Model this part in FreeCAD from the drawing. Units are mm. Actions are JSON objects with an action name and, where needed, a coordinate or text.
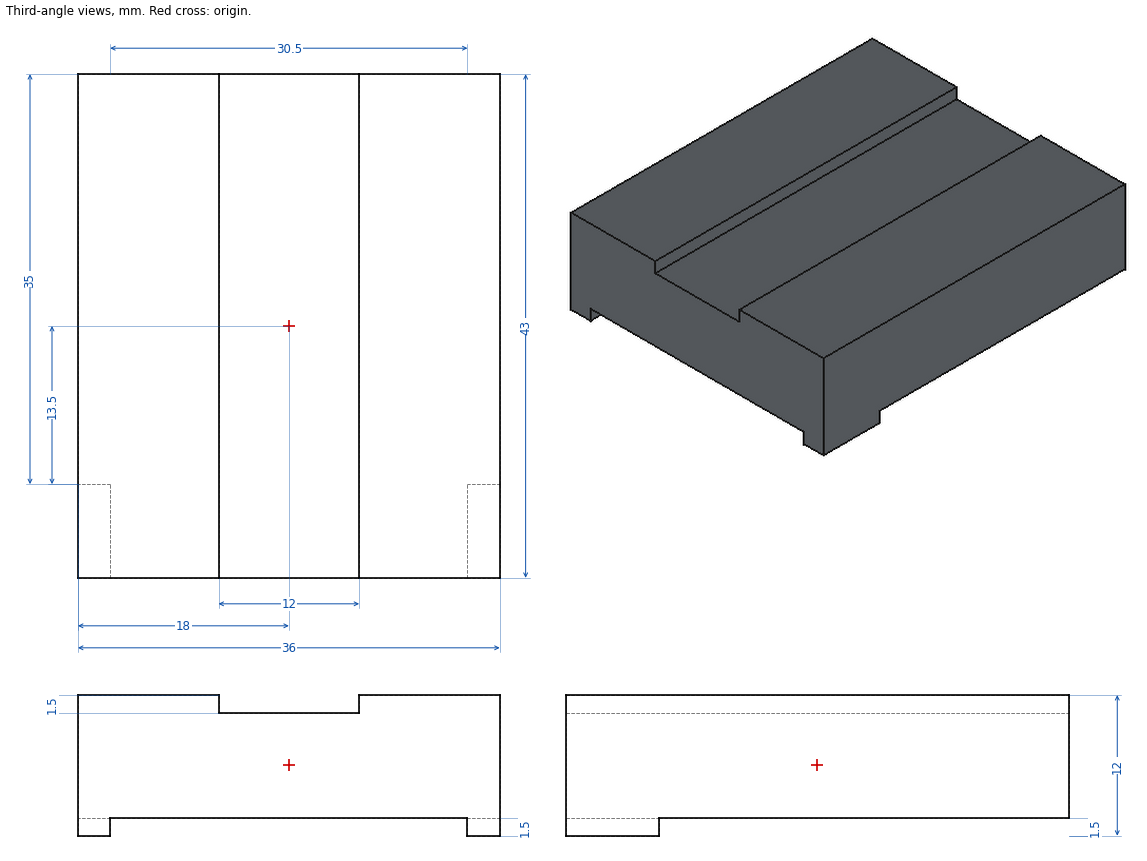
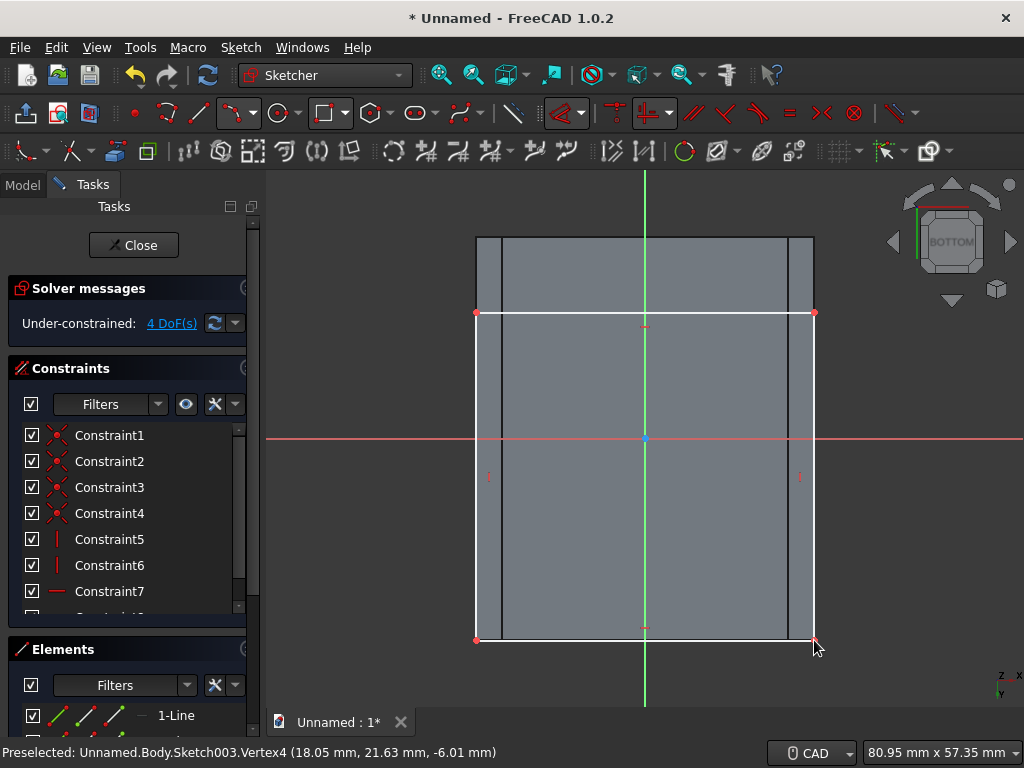
{"action": "key", "text": "d"}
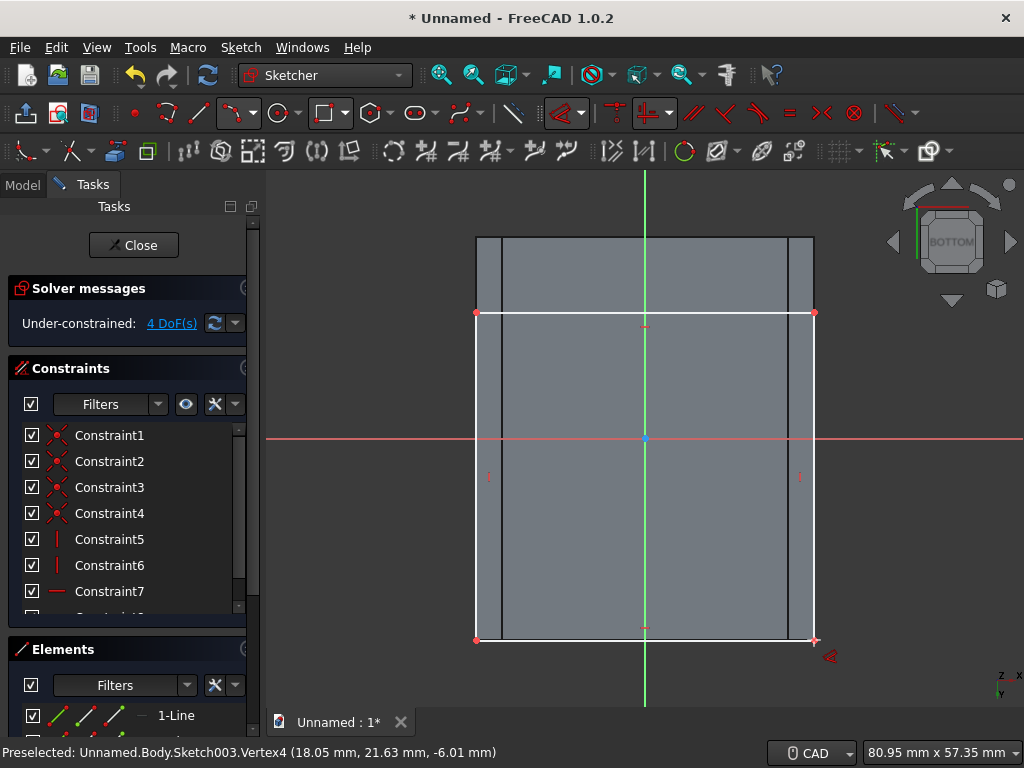
{"action": "left_click", "coordinate": [476, 411]}
{"action": "left_click", "coordinate": [442, 477]}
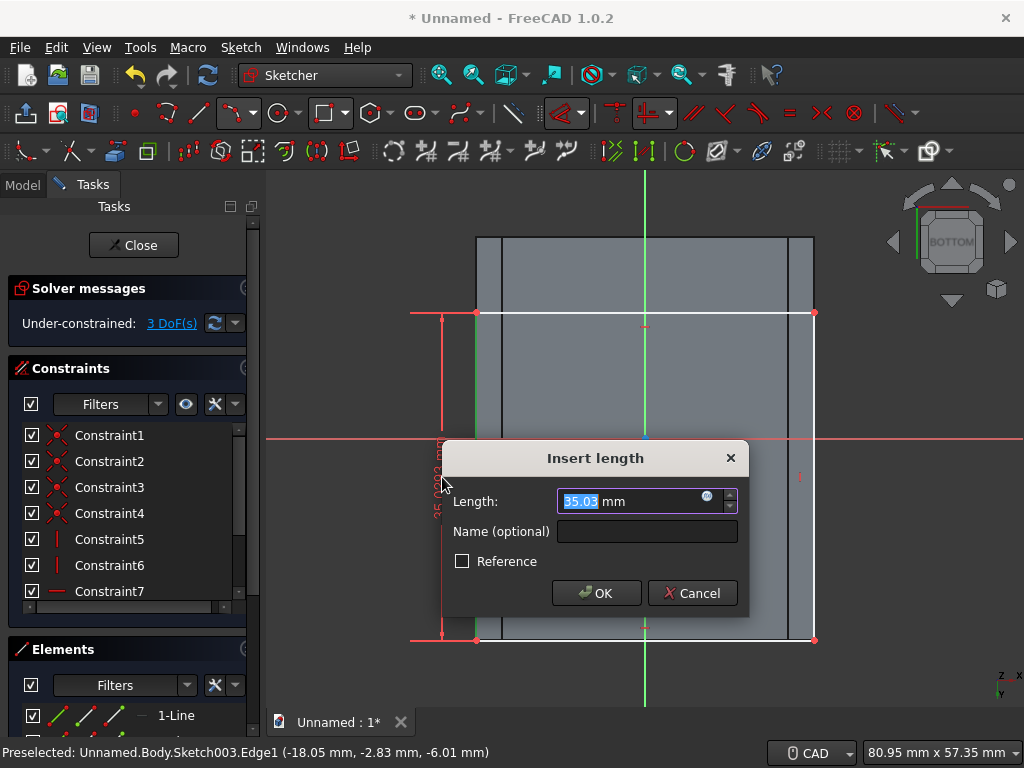
{"action": "type", "text": "35"}
{"action": "key", "text": "Return"}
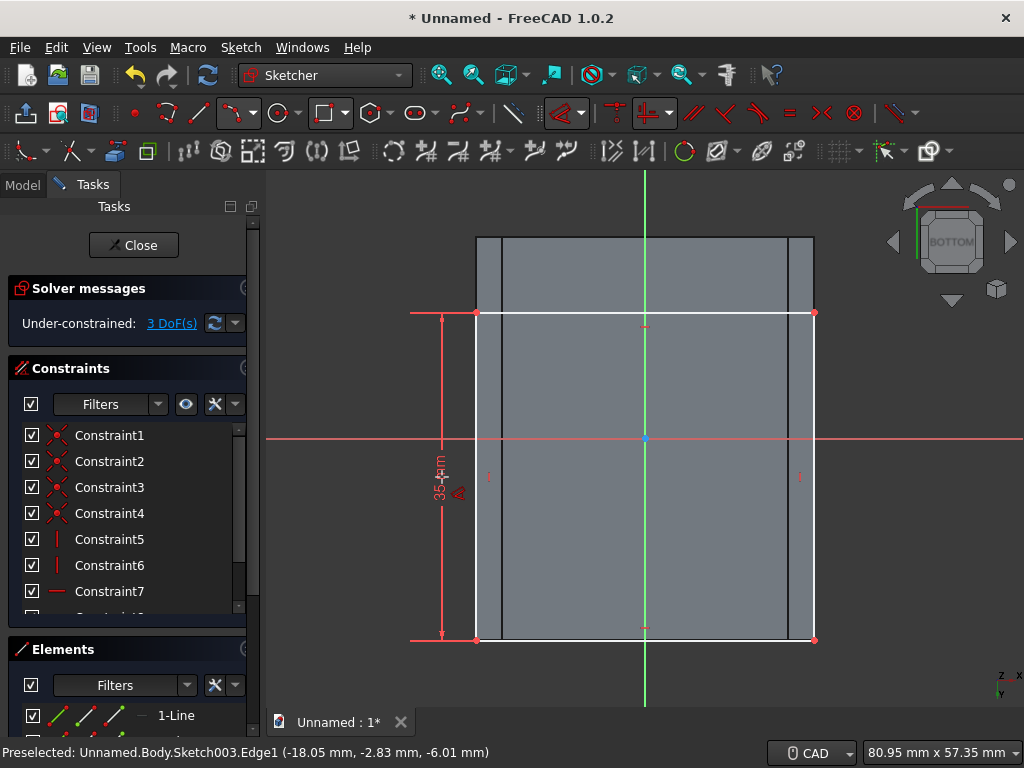
{"action": "left_click", "coordinate": [577, 641]}
{"action": "left_click", "coordinate": [567, 675]}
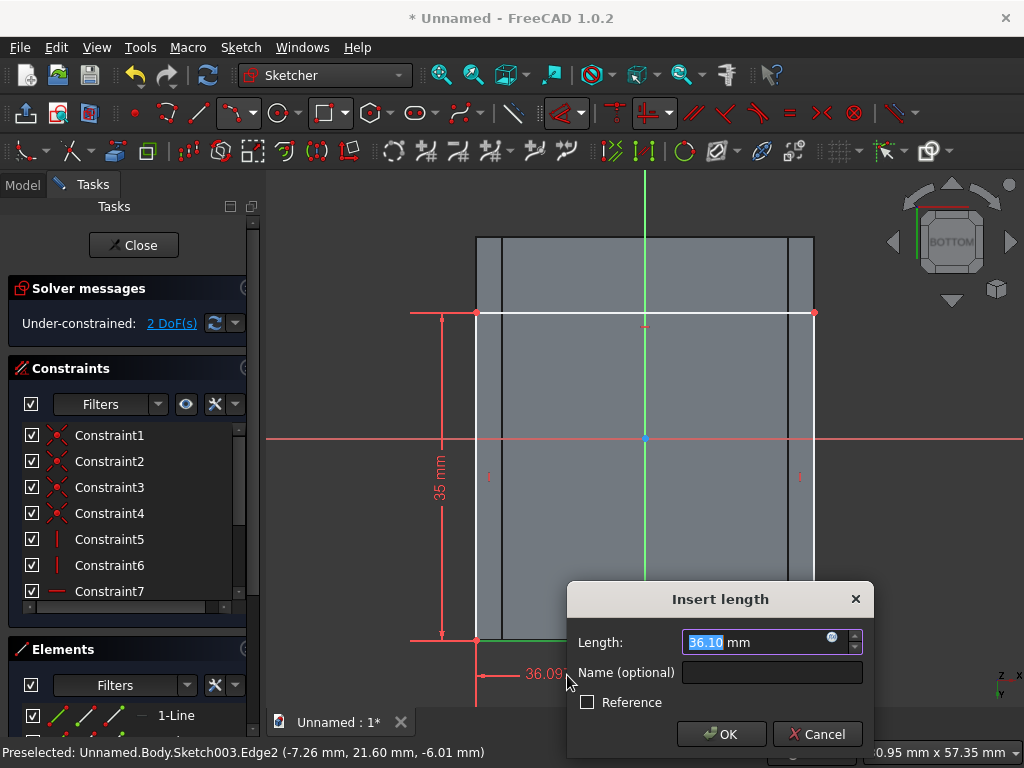
{"action": "type", "text": "36"}
{"action": "key", "text": "Return"}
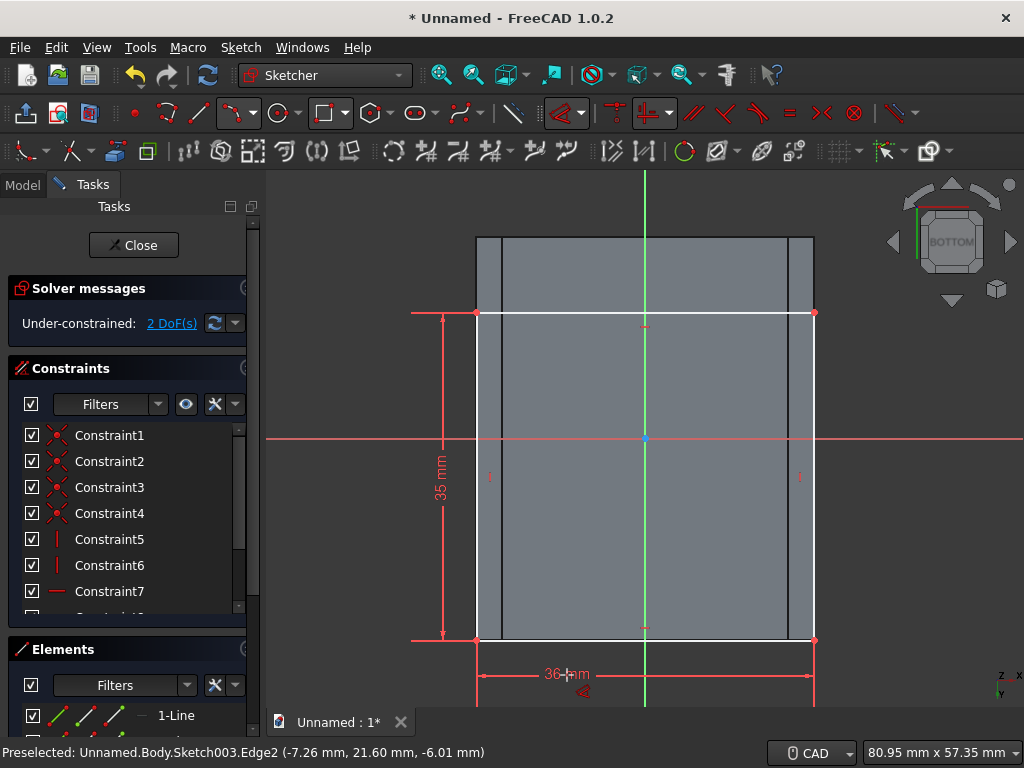
{"action": "left_click", "coordinate": [477, 313]}
{"action": "left_click", "coordinate": [561, 279]}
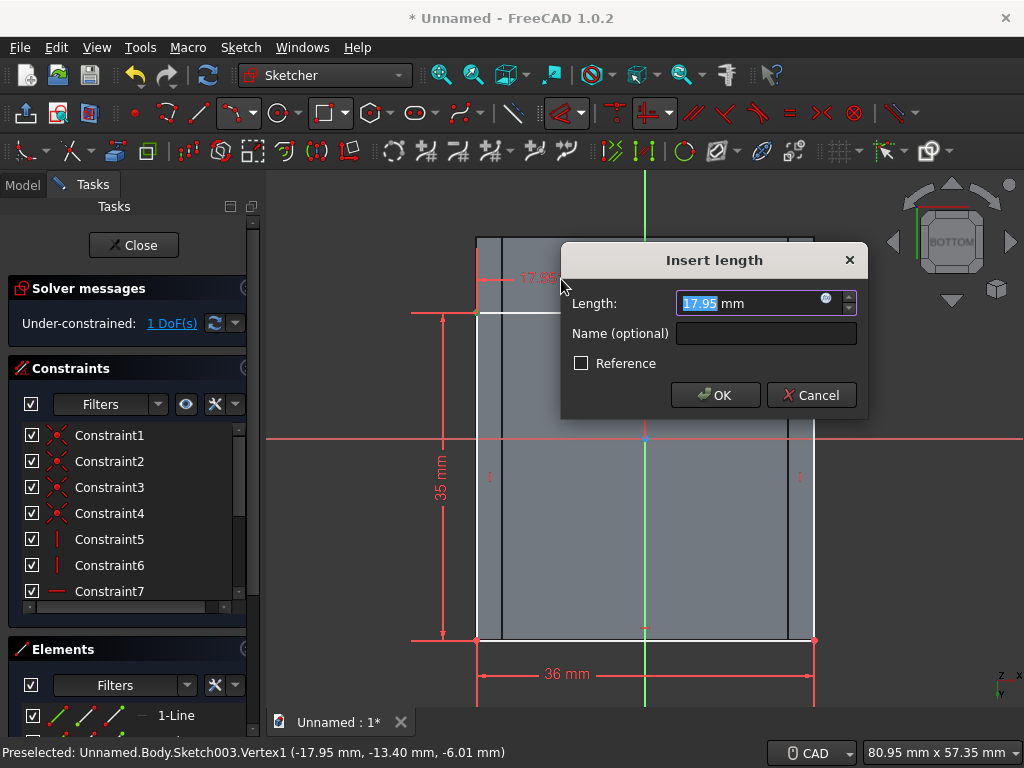
{"action": "type", "text": "18"}
{"action": "key", "text": "Return"}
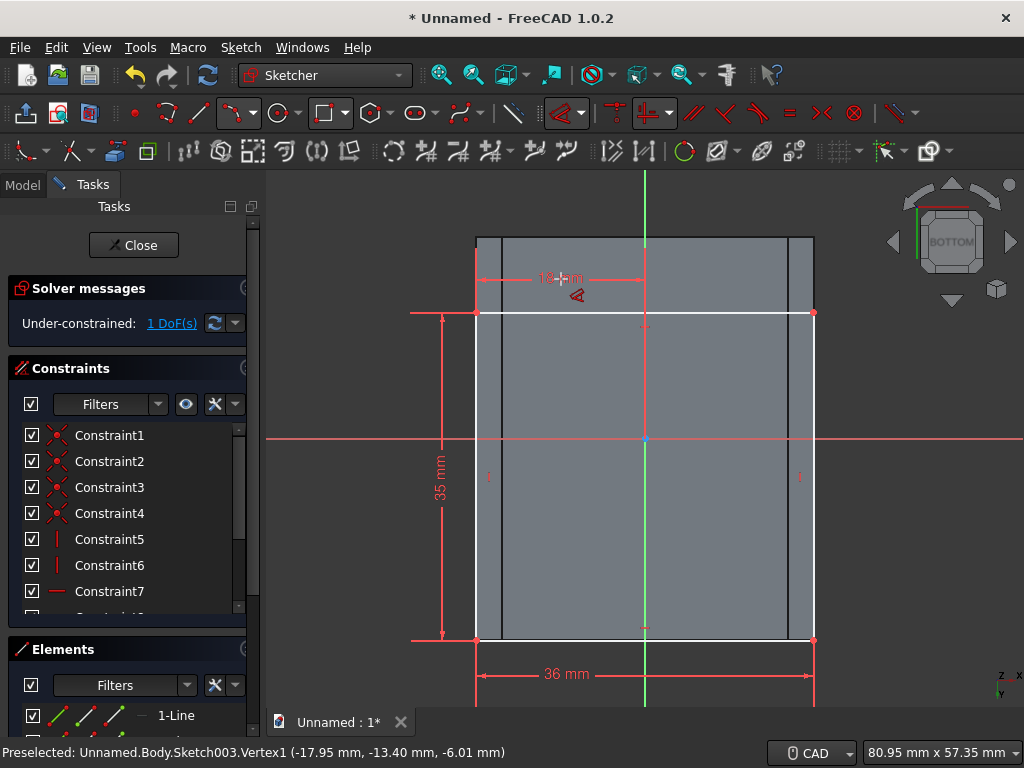
{"action": "left_click", "coordinate": [476, 313]}
{"action": "left_click", "coordinate": [442, 376]}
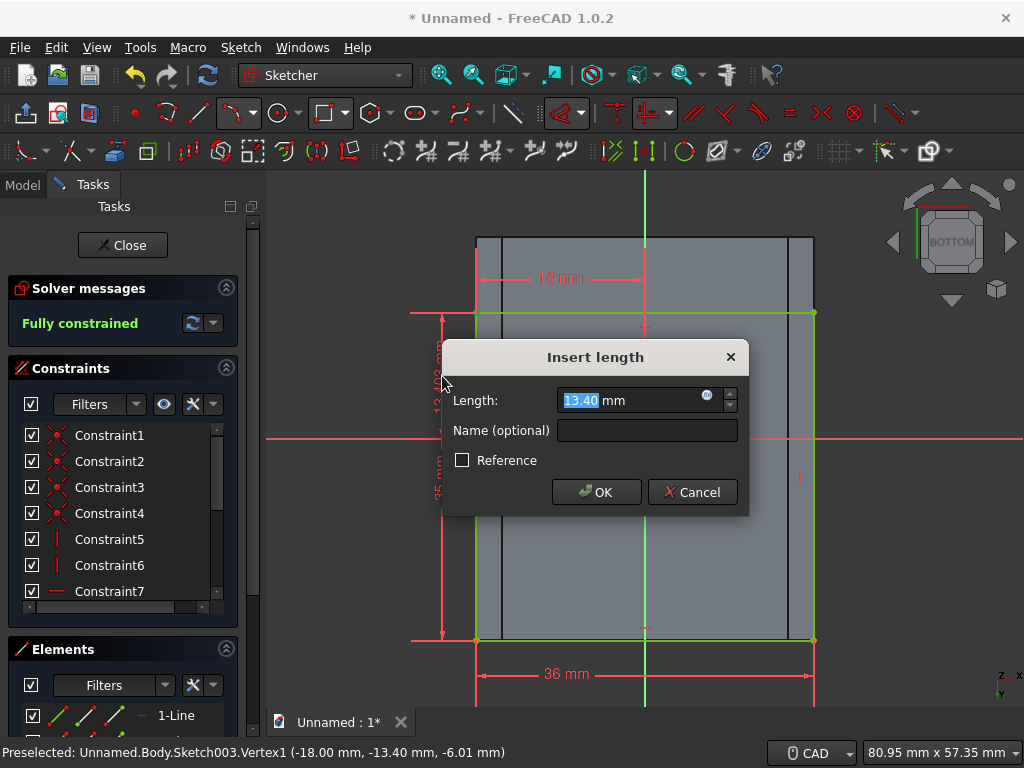
{"action": "type", "text": "13.5"}
{"action": "key", "text": "Return"}
{"action": "key", "text": "Escape"}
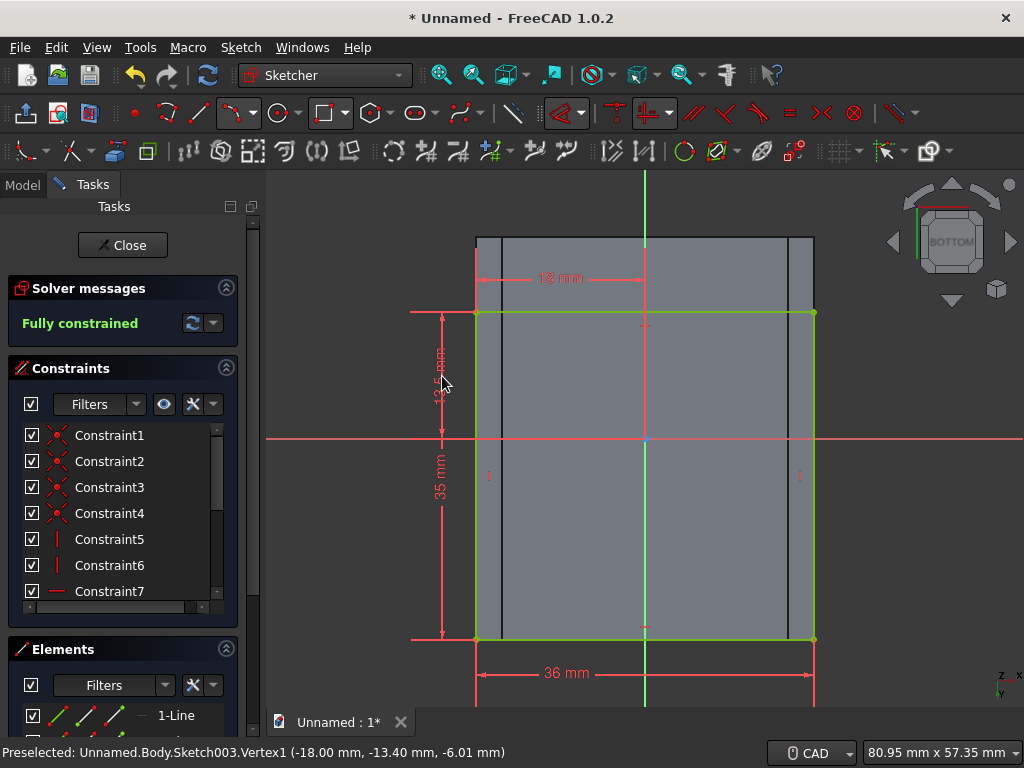
{"action": "left_click", "coordinate": [123, 245]}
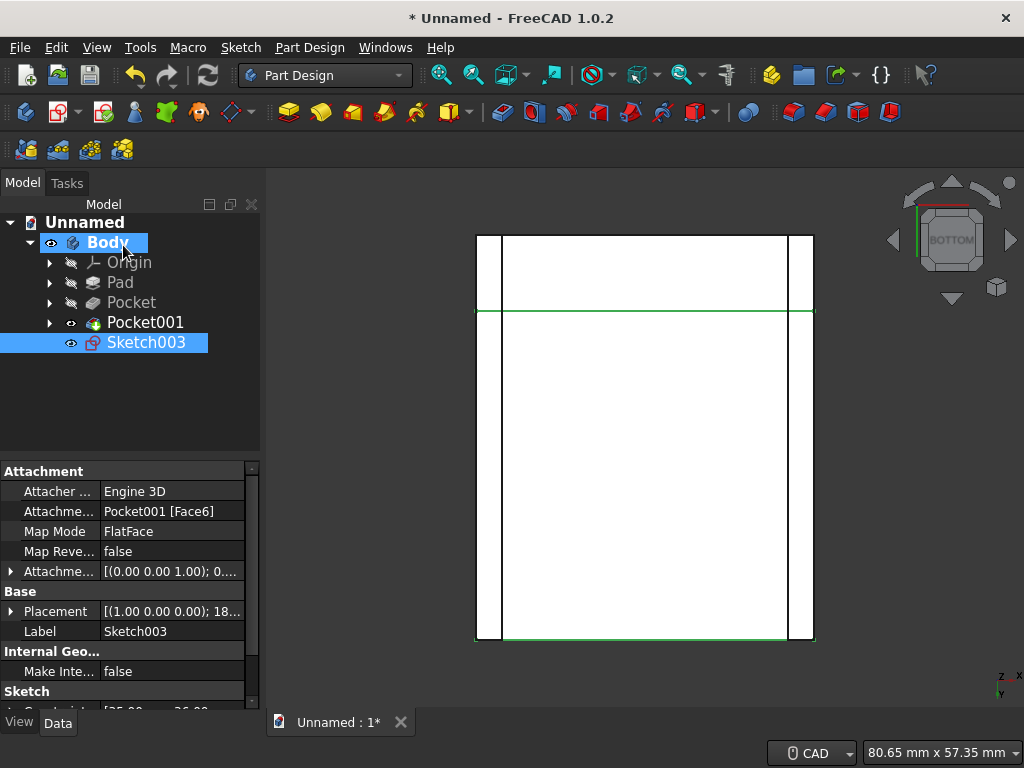
{"action": "left_click", "coordinate": [504, 112]}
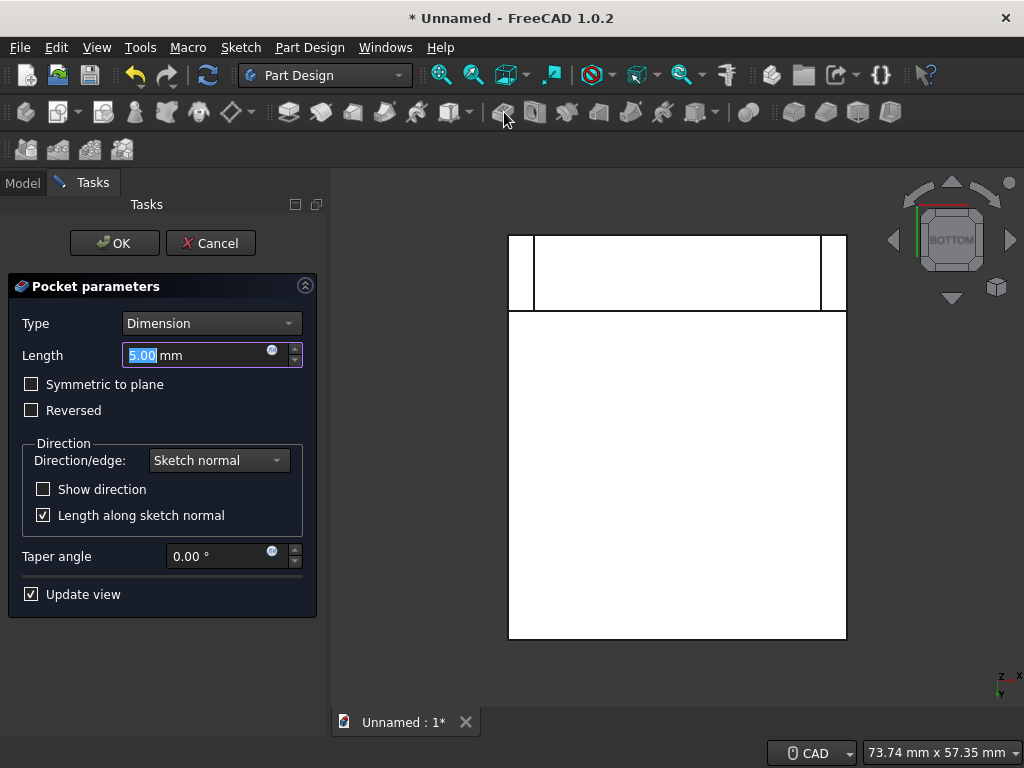
{"action": "type", "text": "1.5"}
{"action": "key", "text": "Tab"}